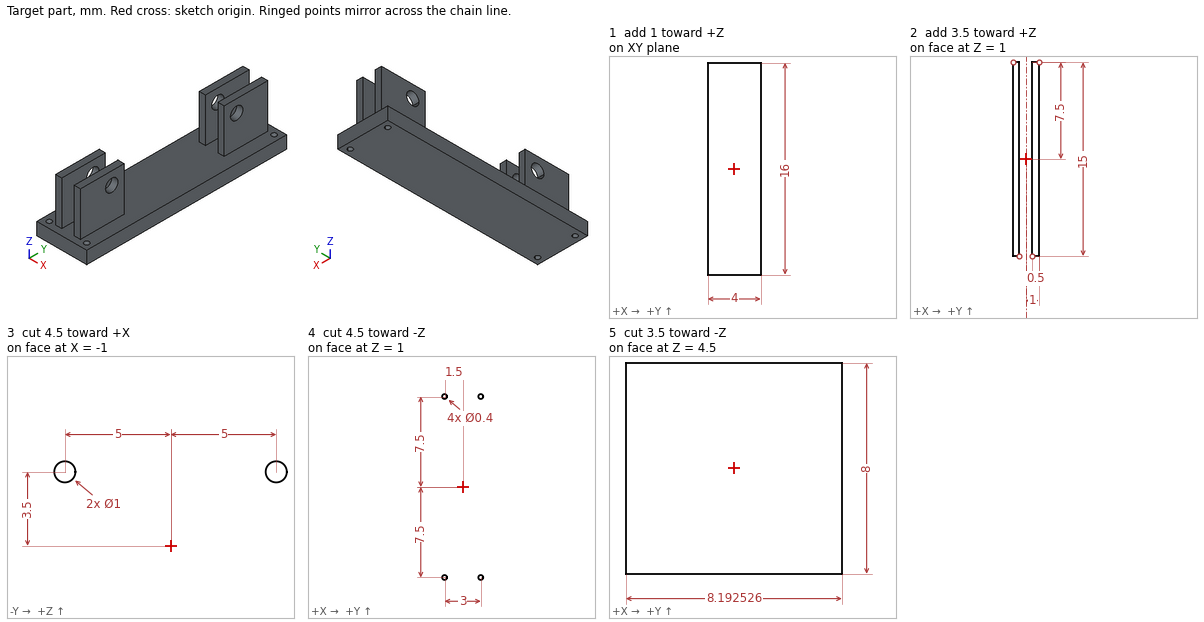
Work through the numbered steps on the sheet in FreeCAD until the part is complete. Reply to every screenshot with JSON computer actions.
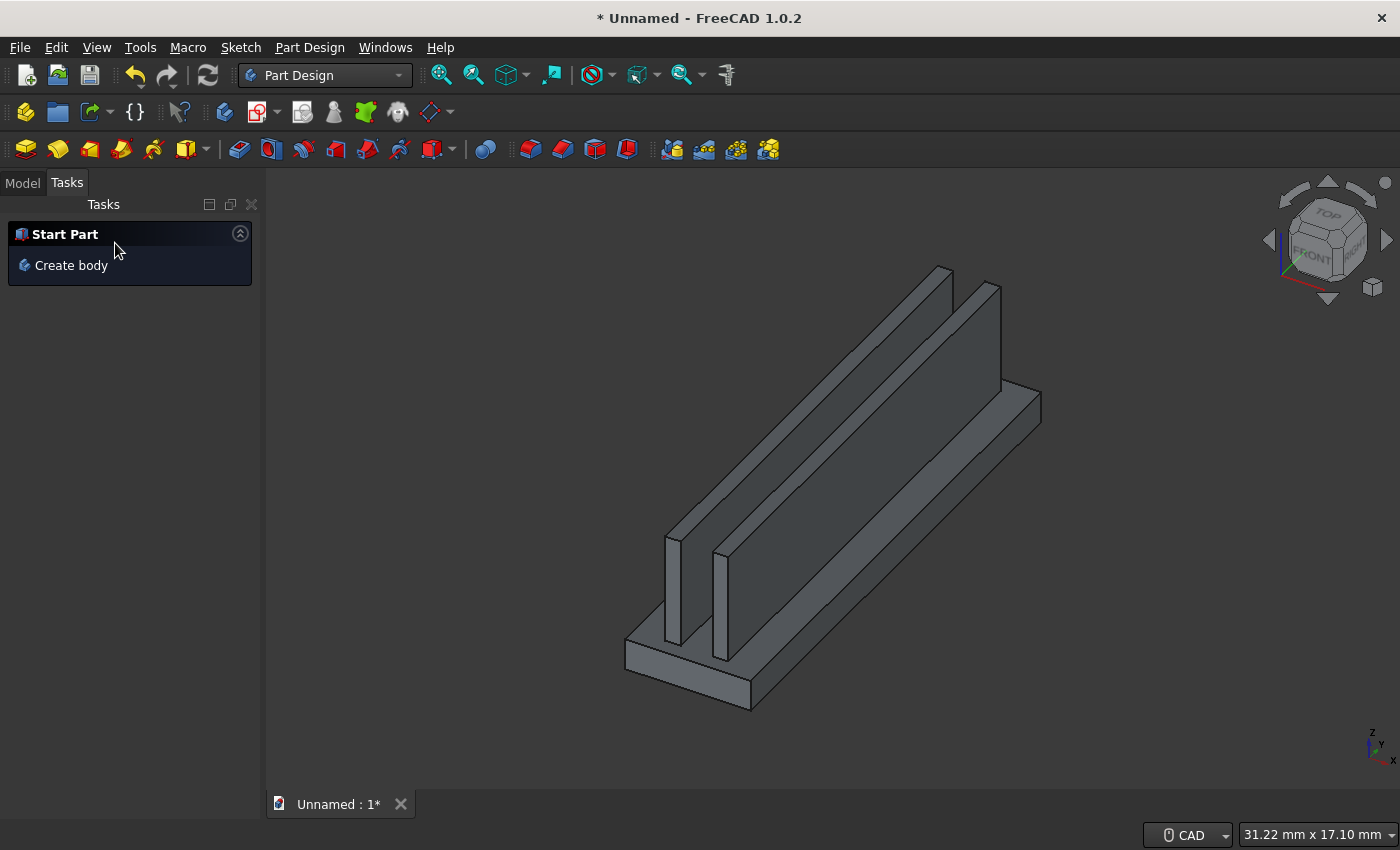
{"action": "key", "text": "6"}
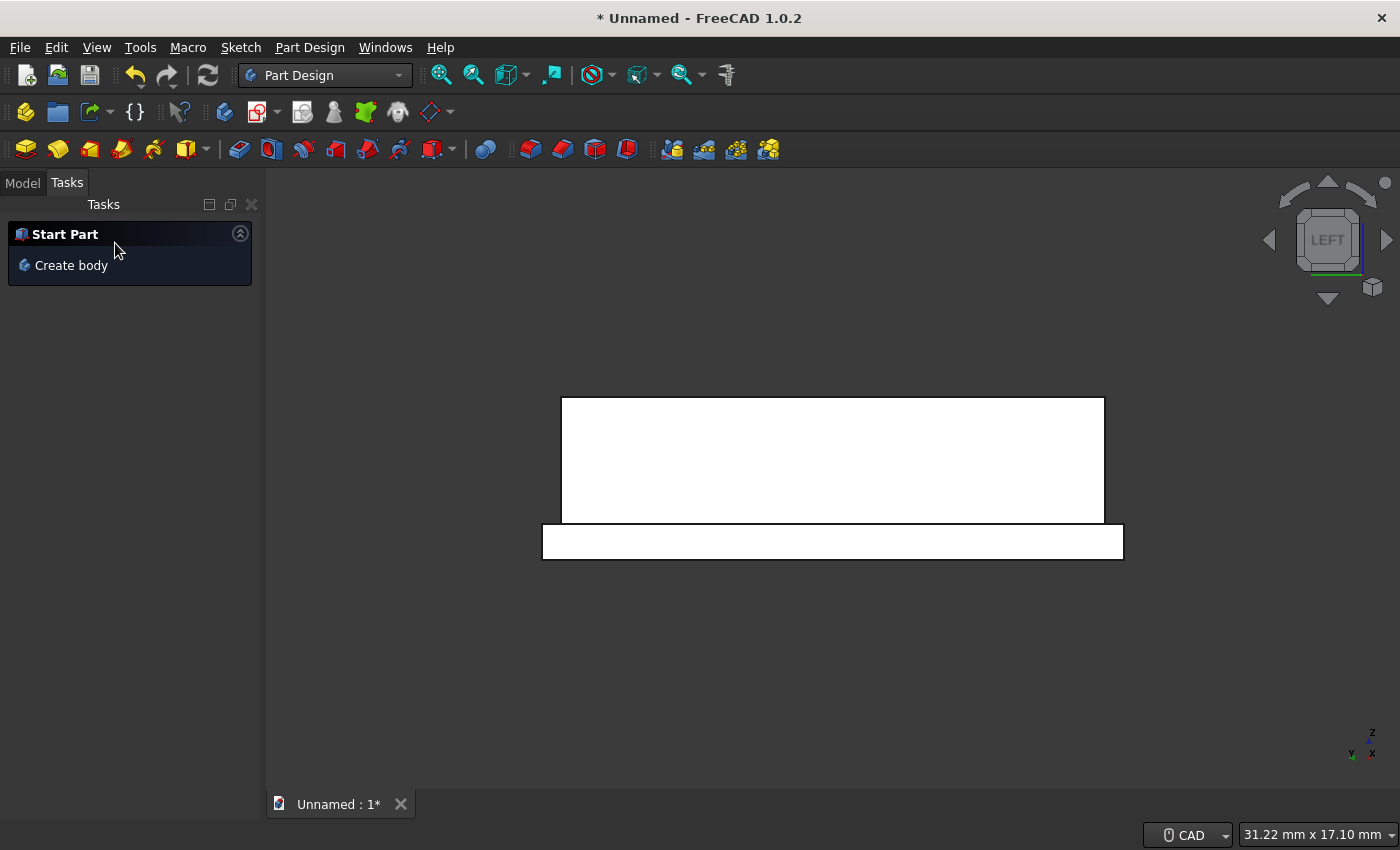
{"action": "left_click", "coordinate": [677, 459]}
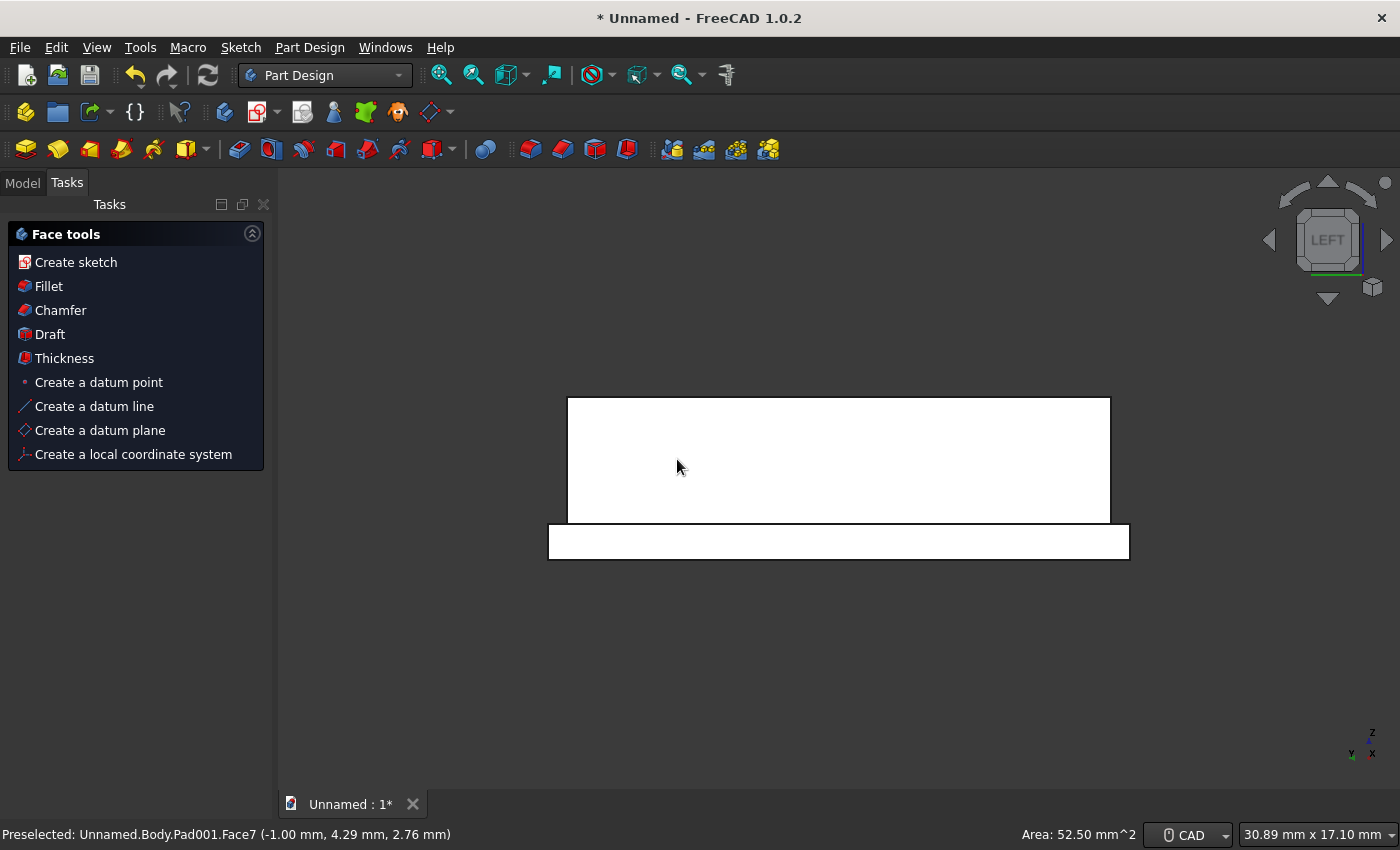
{"action": "left_click", "coordinate": [258, 112]}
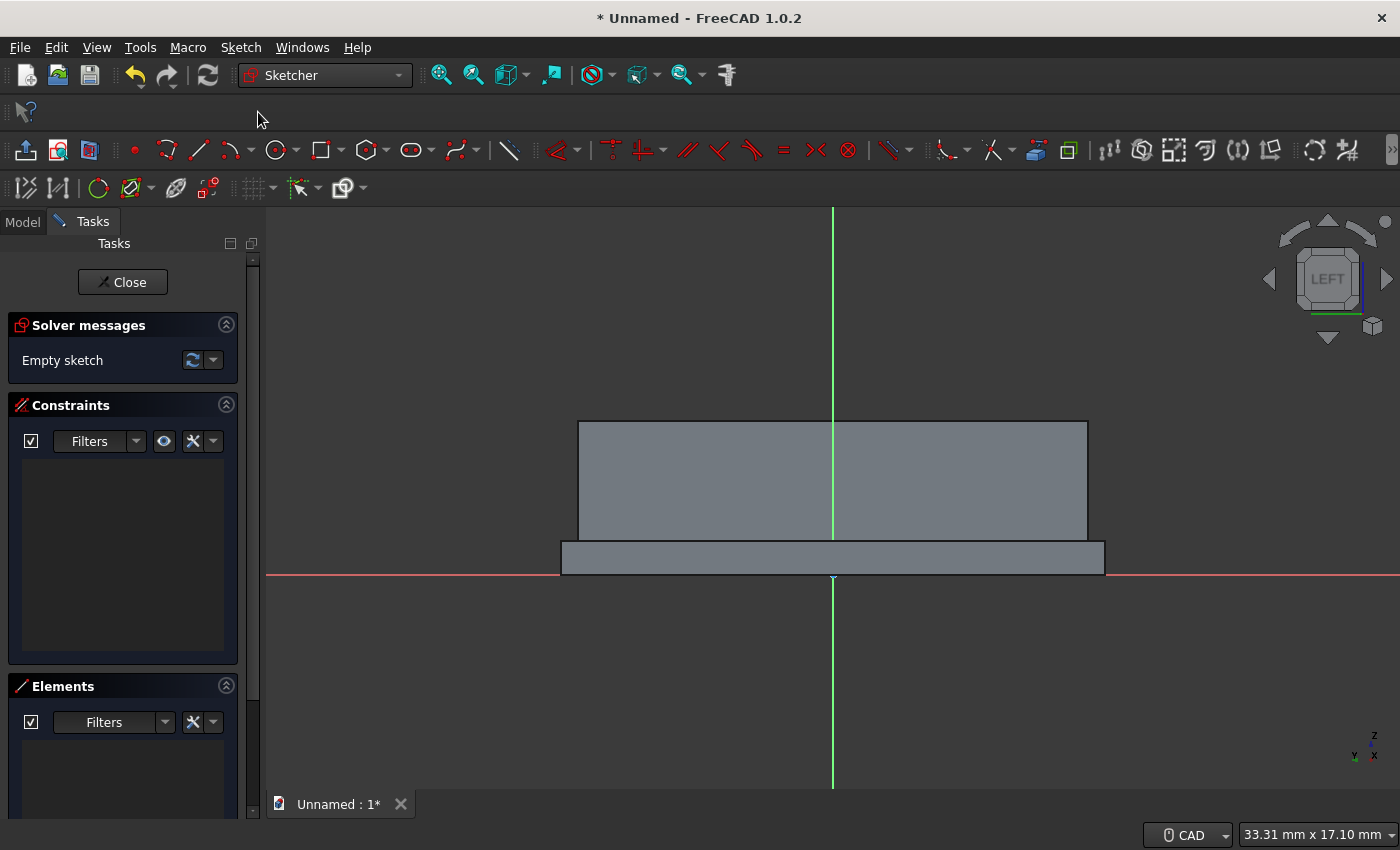
{"action": "scroll", "coordinate": [916, 517], "scroll_direction": "up", "scroll_amount": 3}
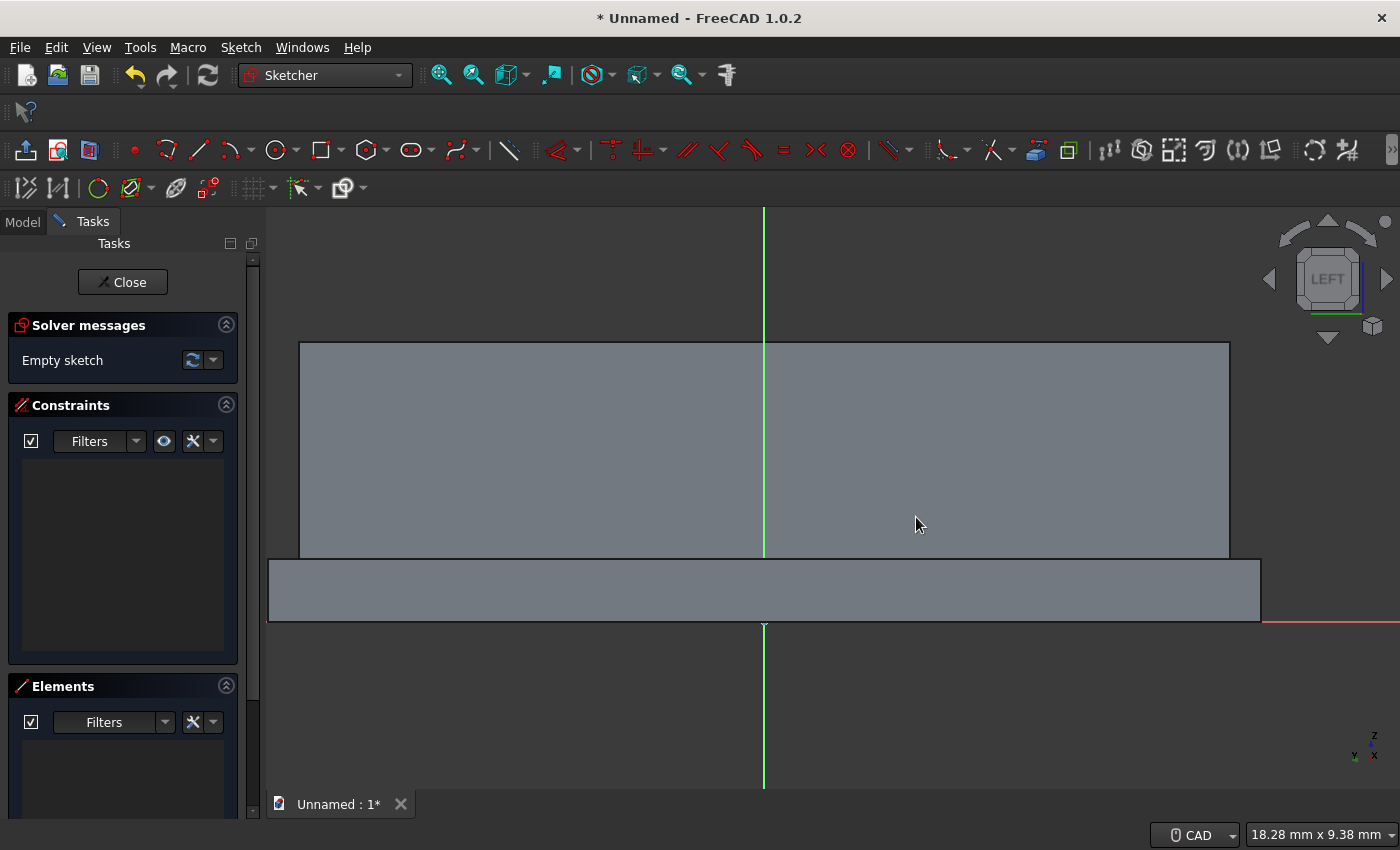
{"action": "left_click", "coordinate": [276, 150]}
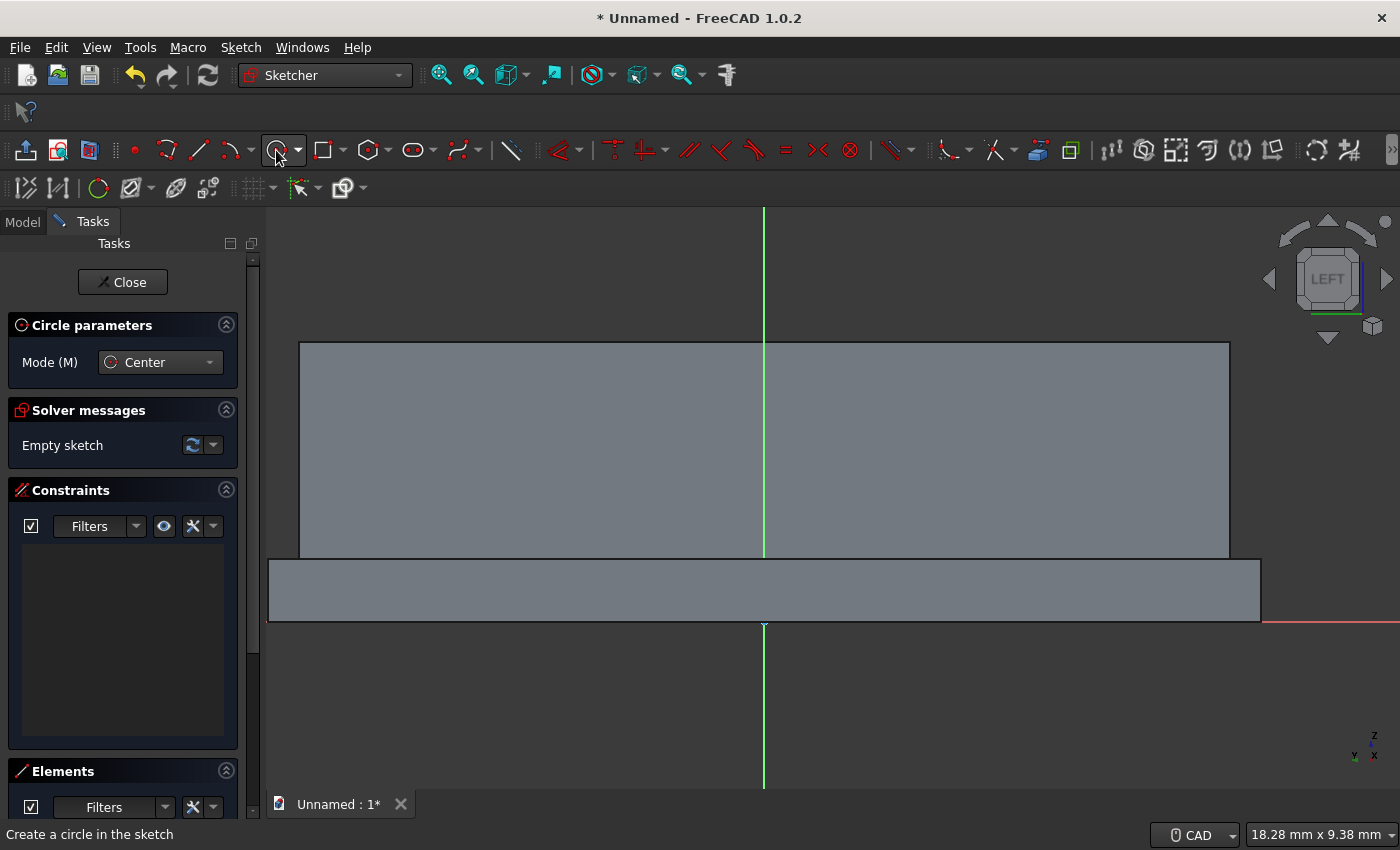
{"action": "left_click", "coordinate": [454, 404]}
{"action": "left_click", "coordinate": [476, 382]}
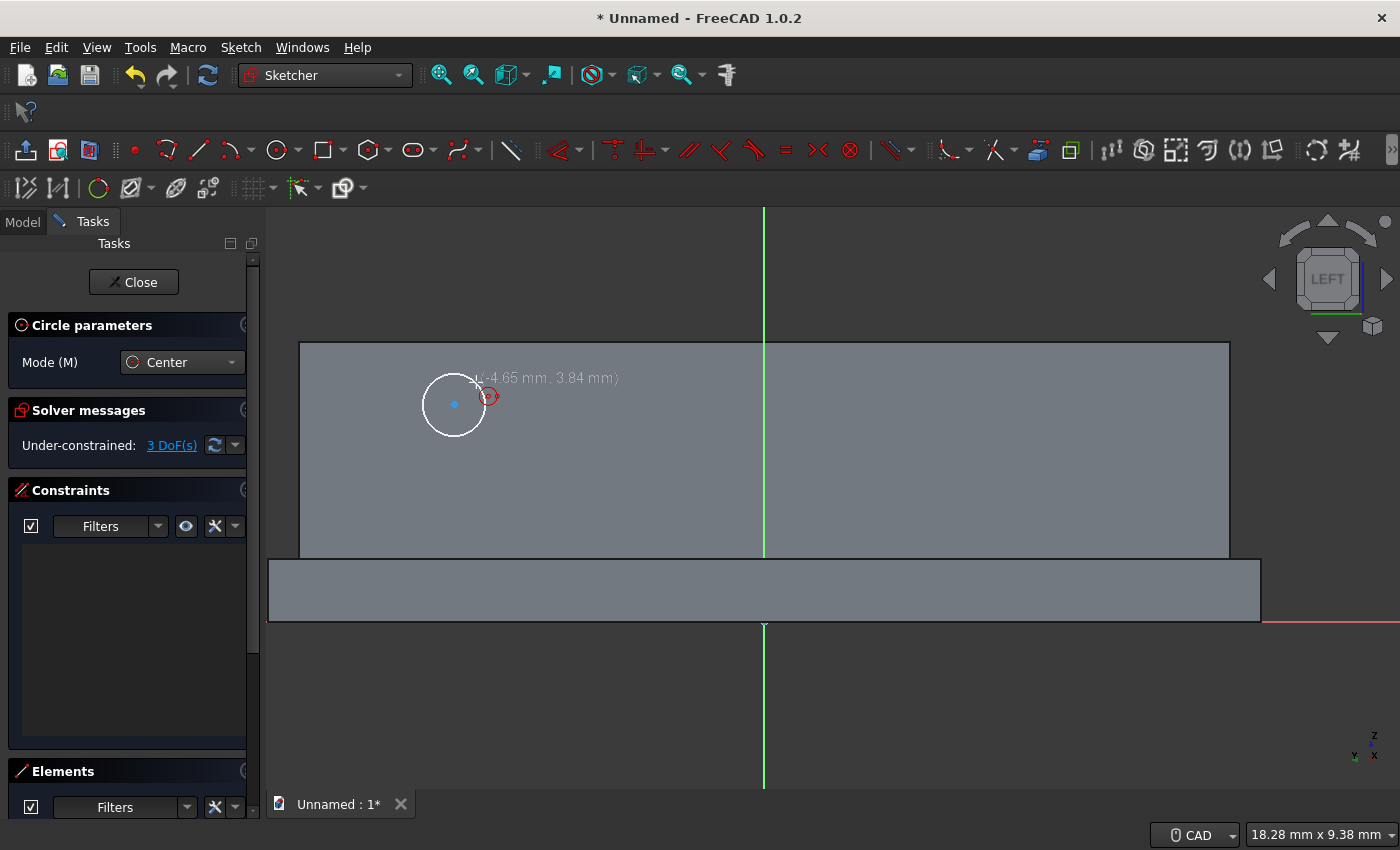
{"action": "left_click", "coordinate": [1074, 404]}
{"action": "left_click", "coordinate": [1096, 382]}
{"action": "key", "text": "Escape"}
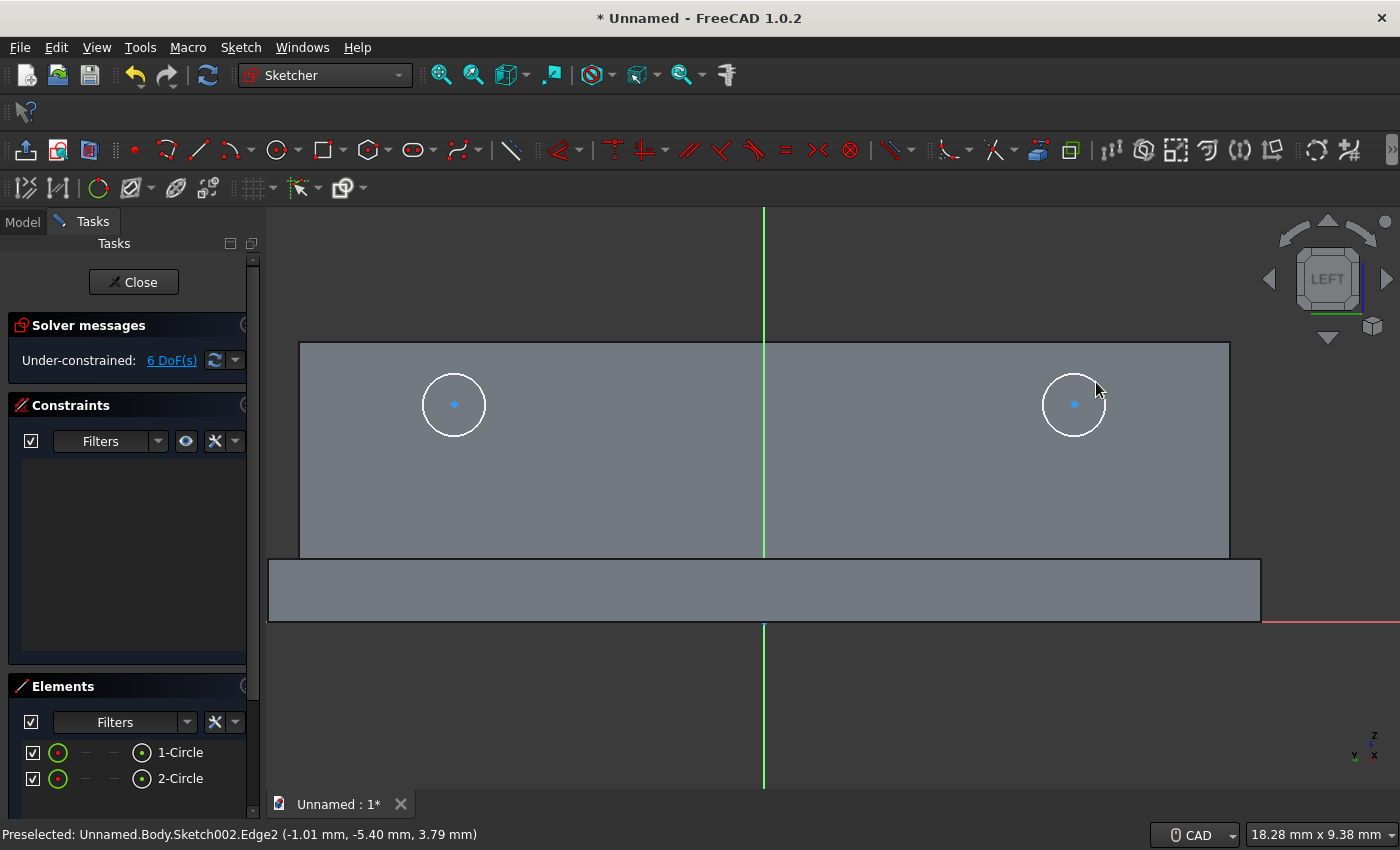
{"action": "left_click", "coordinate": [476, 383]}